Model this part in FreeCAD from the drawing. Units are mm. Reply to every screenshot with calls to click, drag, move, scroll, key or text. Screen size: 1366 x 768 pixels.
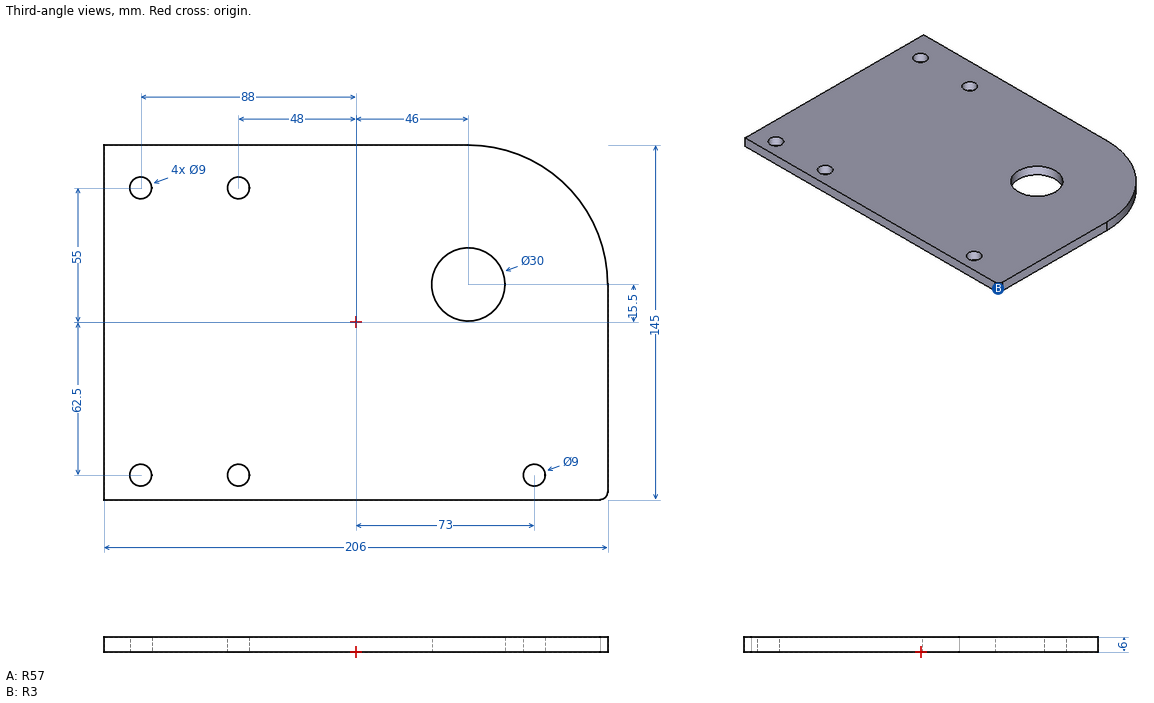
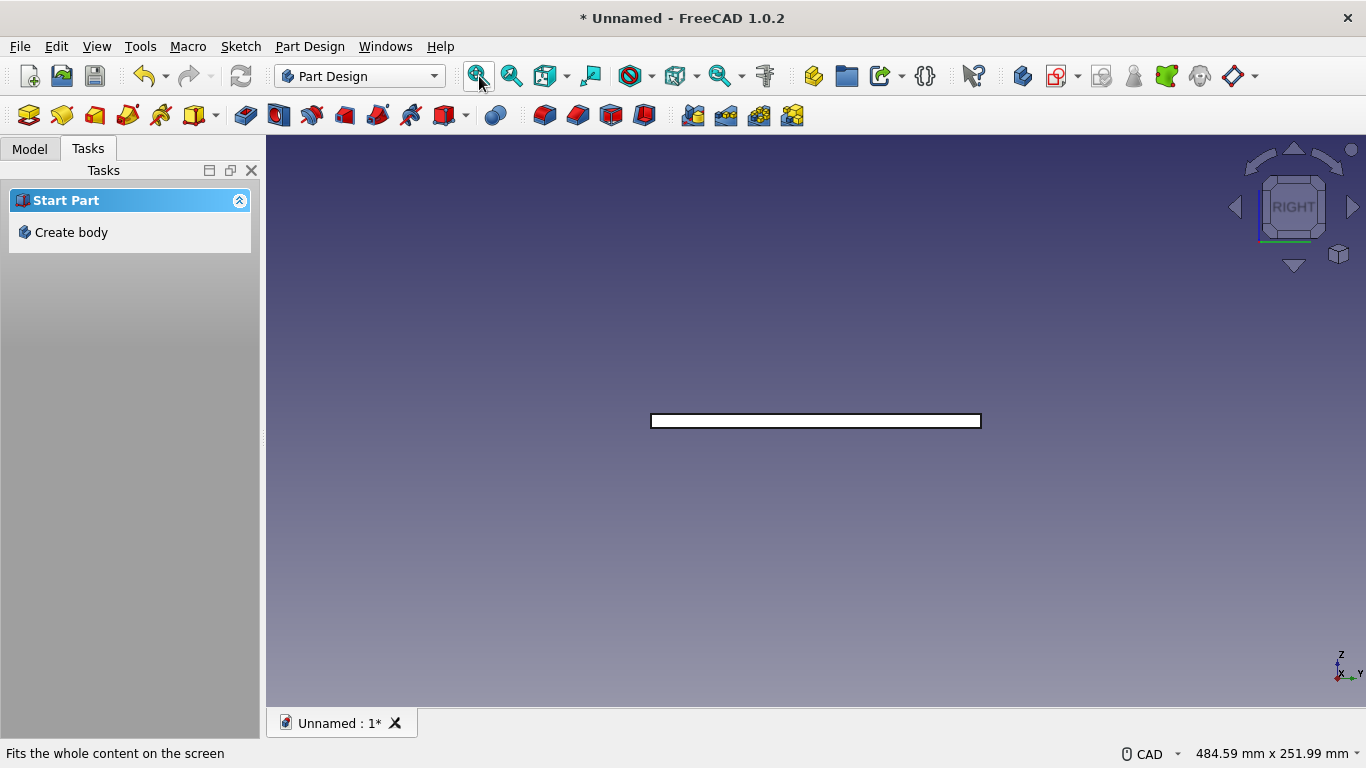
click(981, 420)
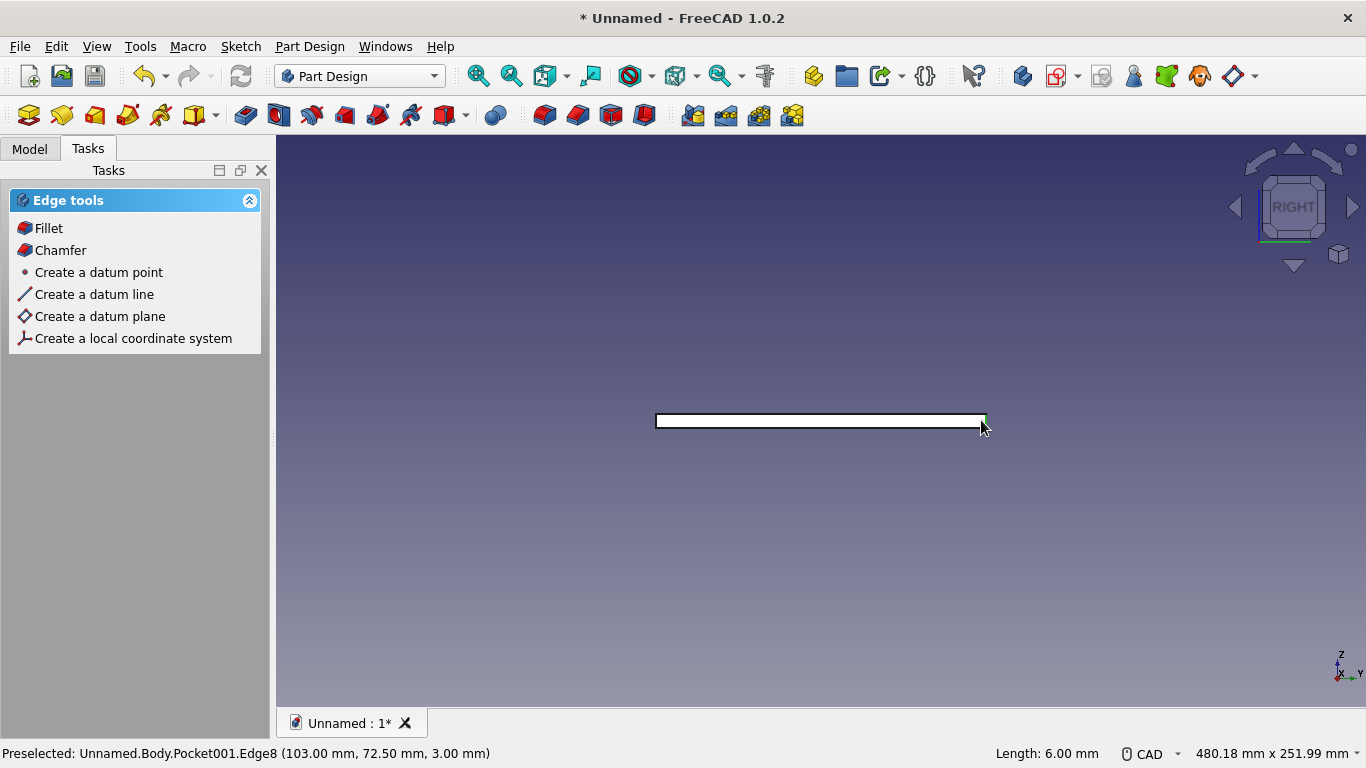
click(545, 116)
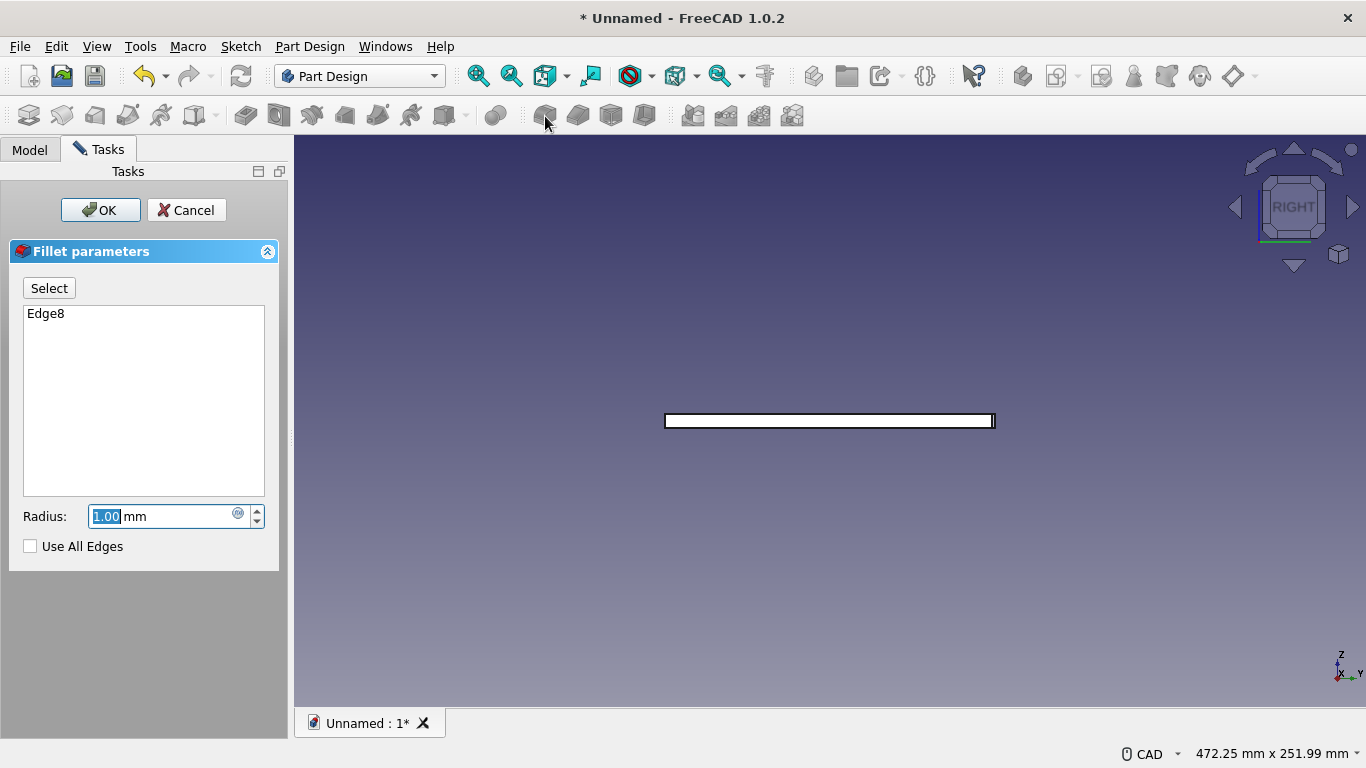
text(57)
key(Tab)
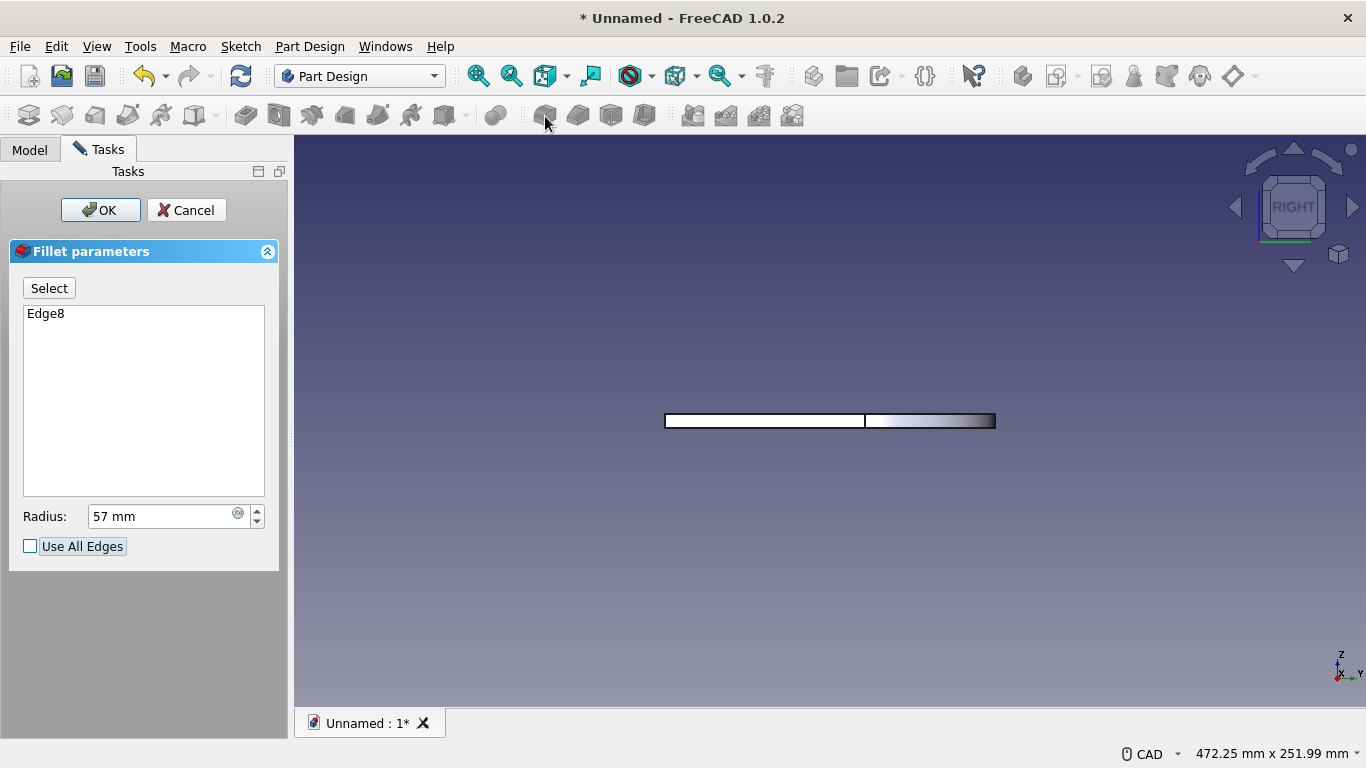
click(101, 210)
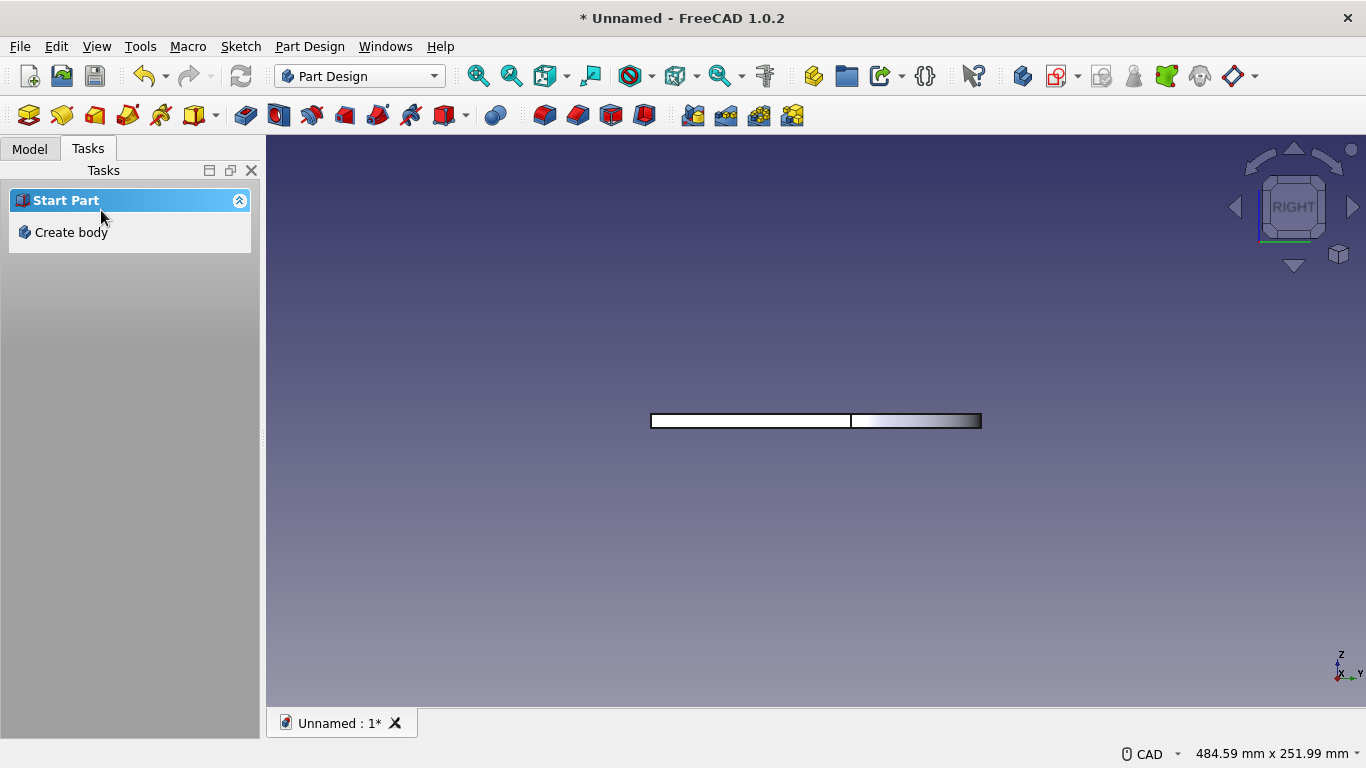
click(479, 76)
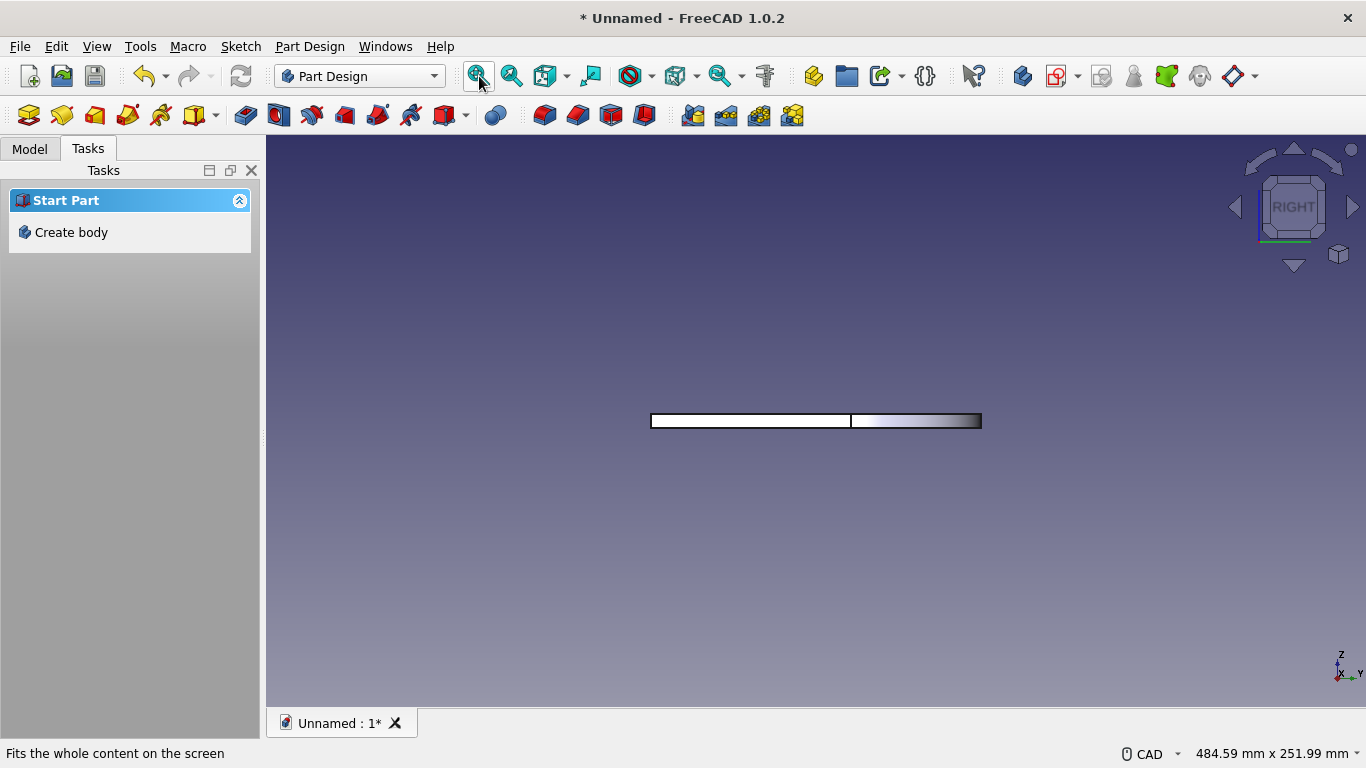
key(0)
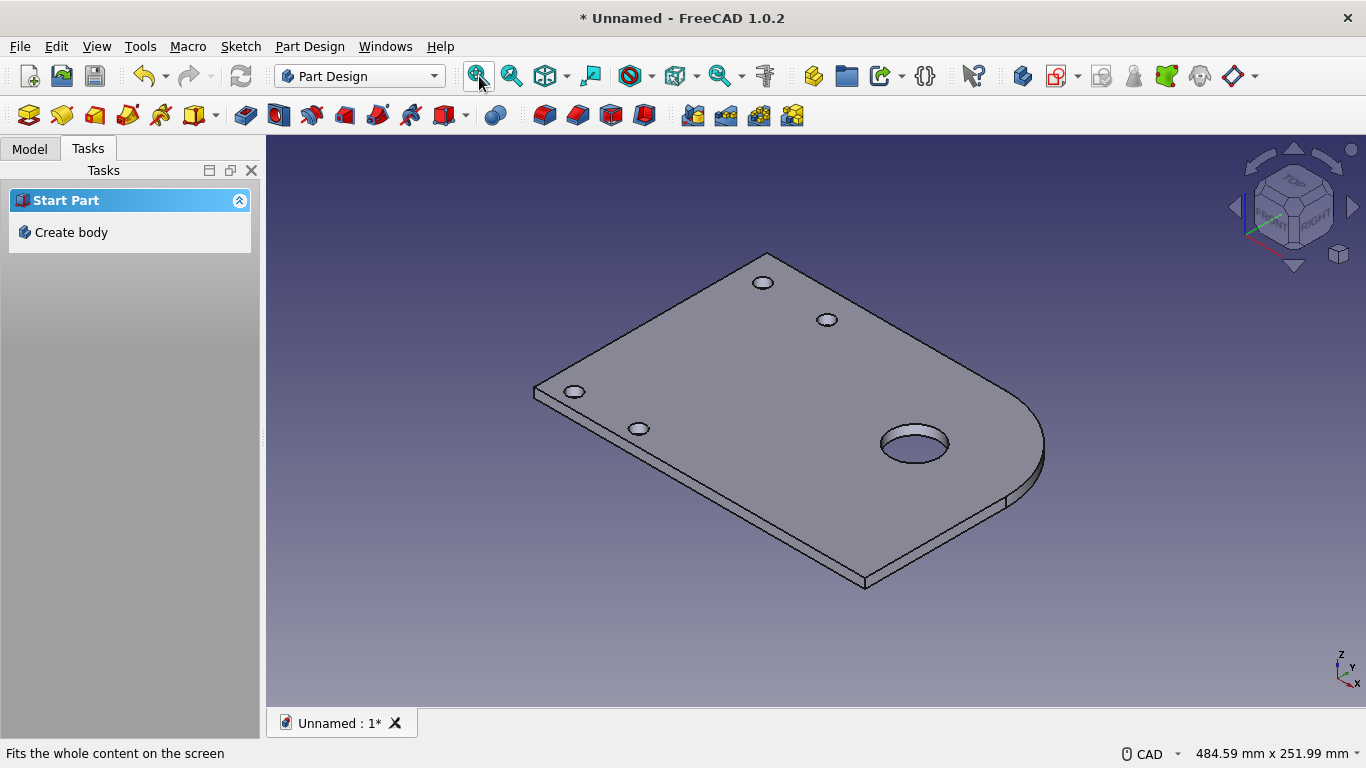
click(769, 387)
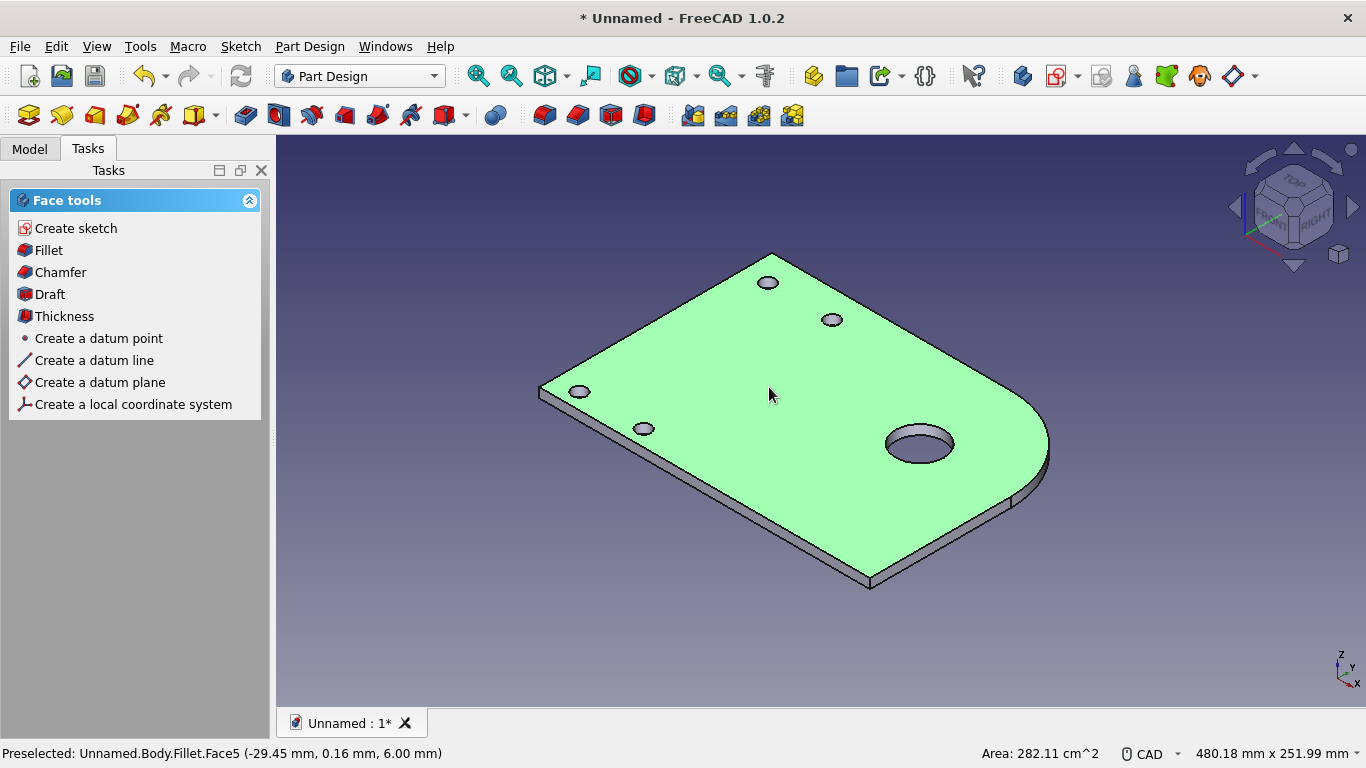
click(1056, 76)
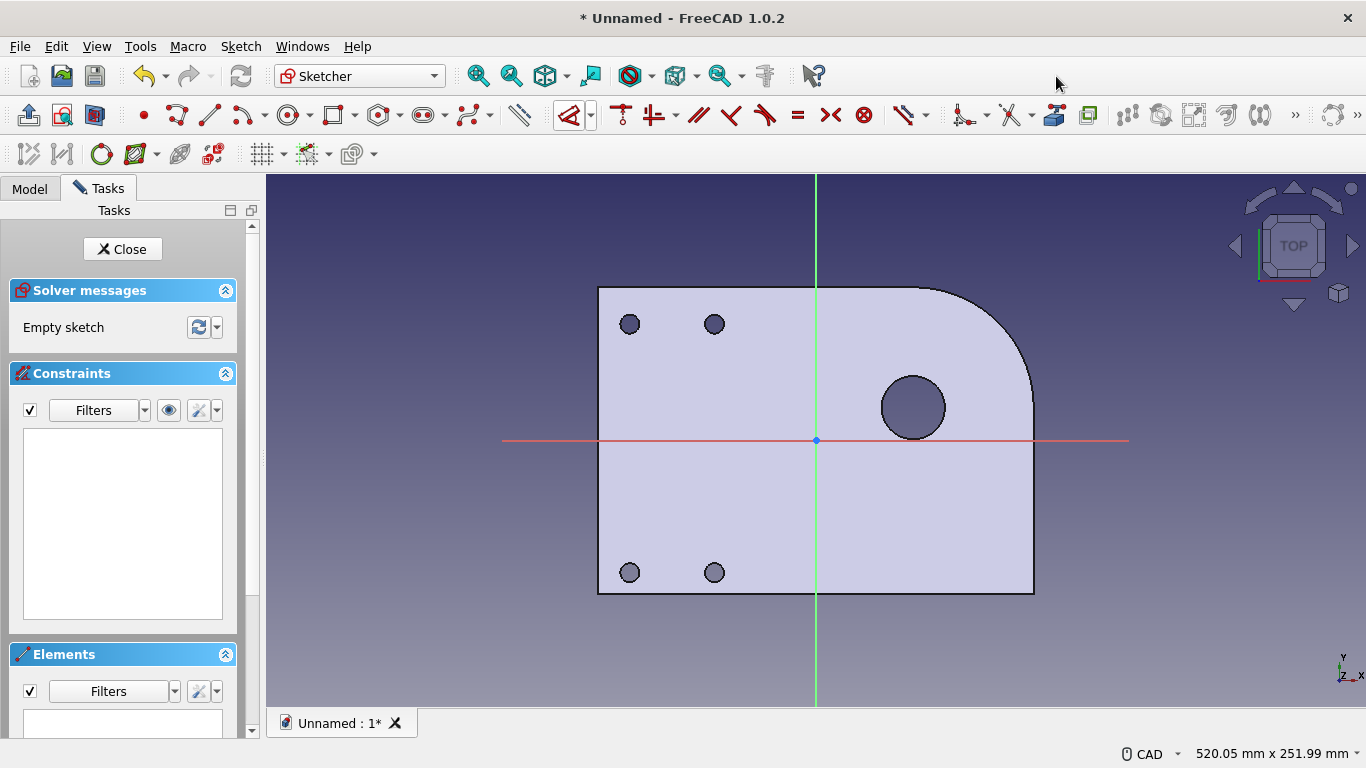
scroll(985, 581, up, 14)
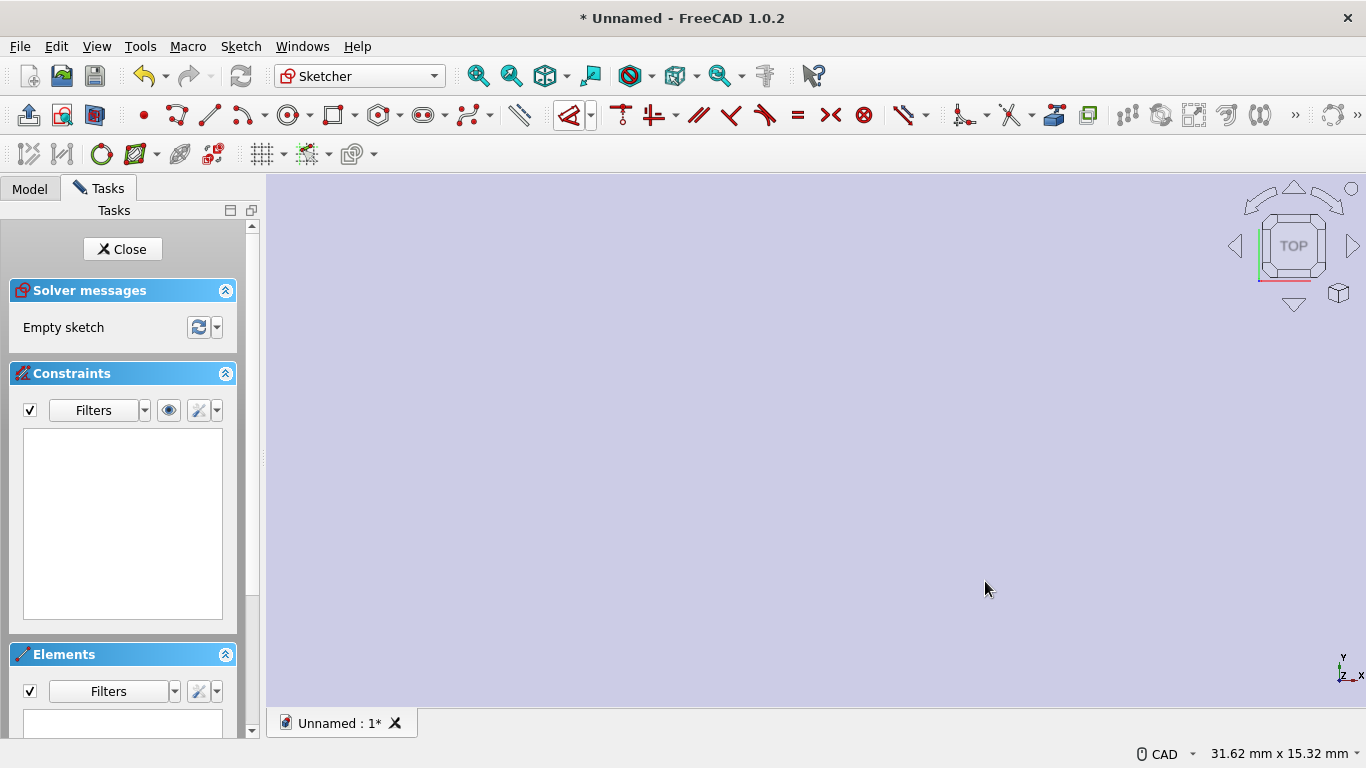
click(288, 116)